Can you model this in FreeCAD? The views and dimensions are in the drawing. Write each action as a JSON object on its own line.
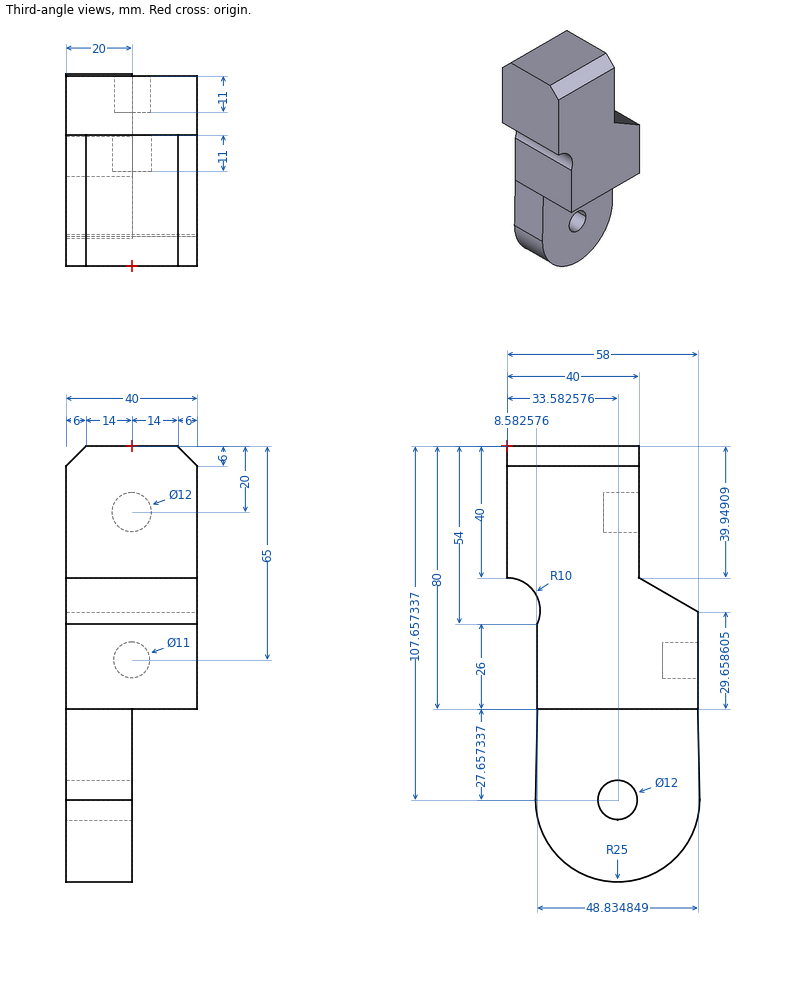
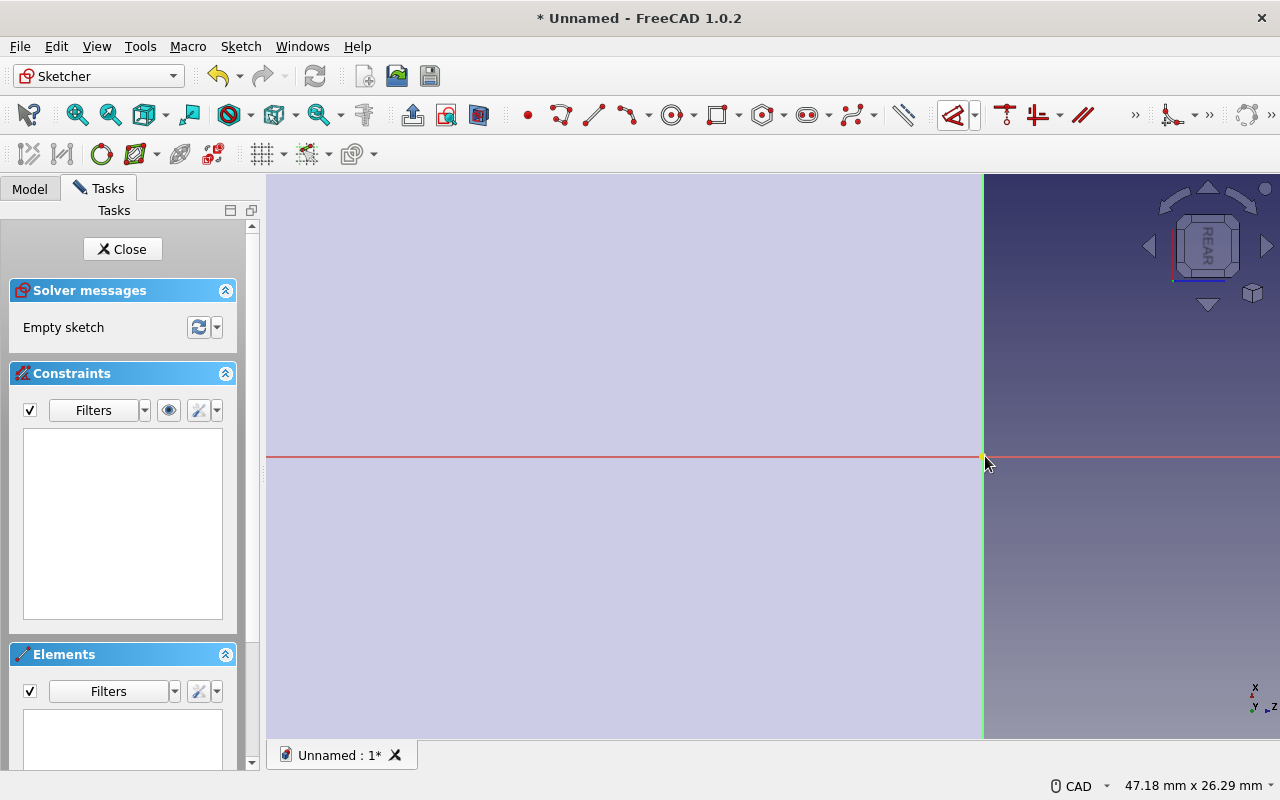
{"action": "key", "text": "g c"}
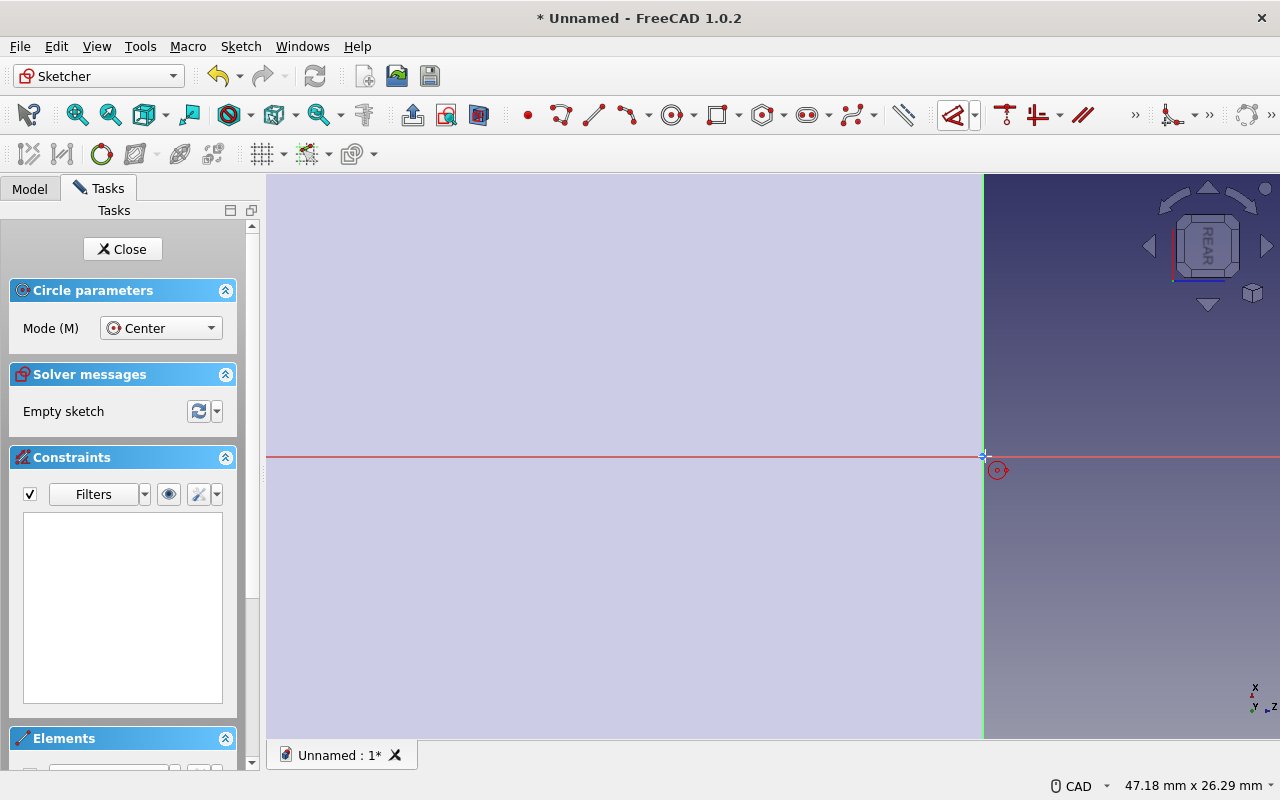
{"action": "left_click", "coordinate": [553, 456]}
{"action": "mouse_move", "coordinate": [644, 365]}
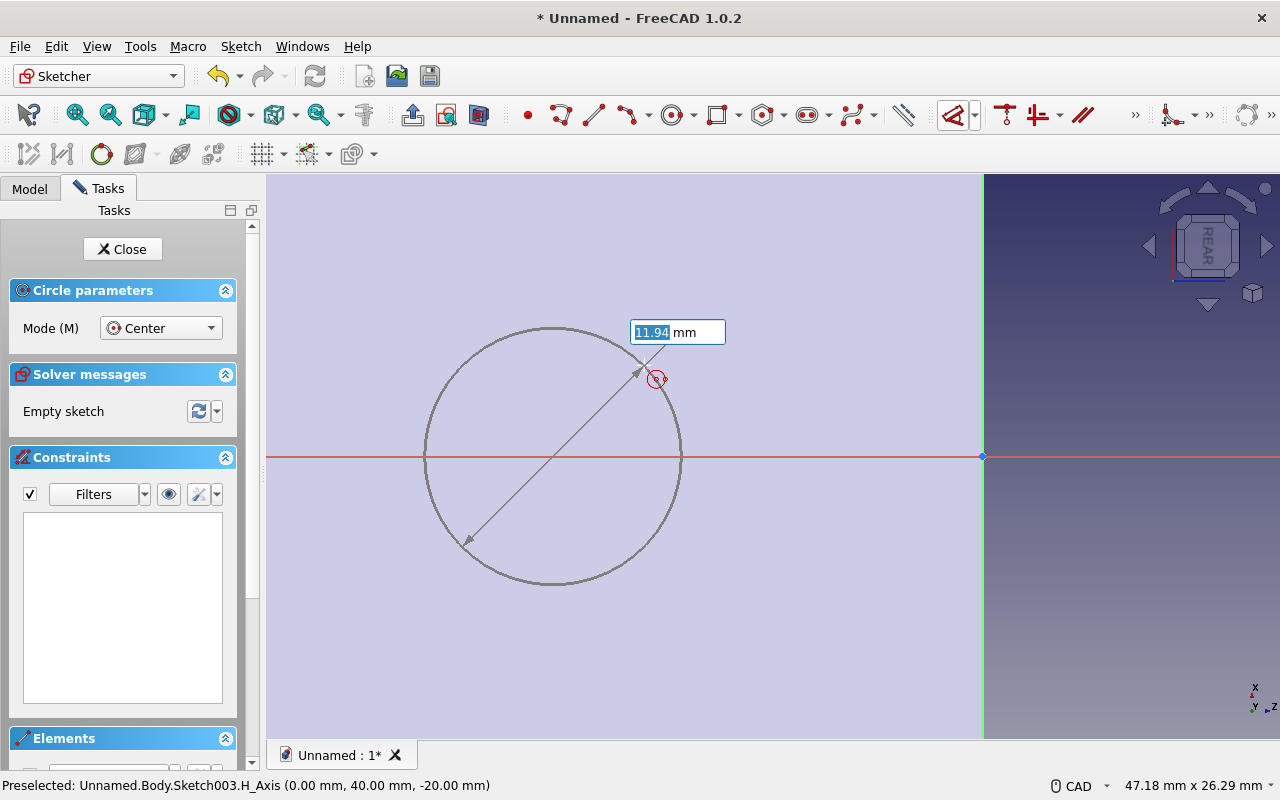
{"action": "type", "text": "12"}
{"action": "key", "text": "Return"}
{"action": "key", "text": "Escape"}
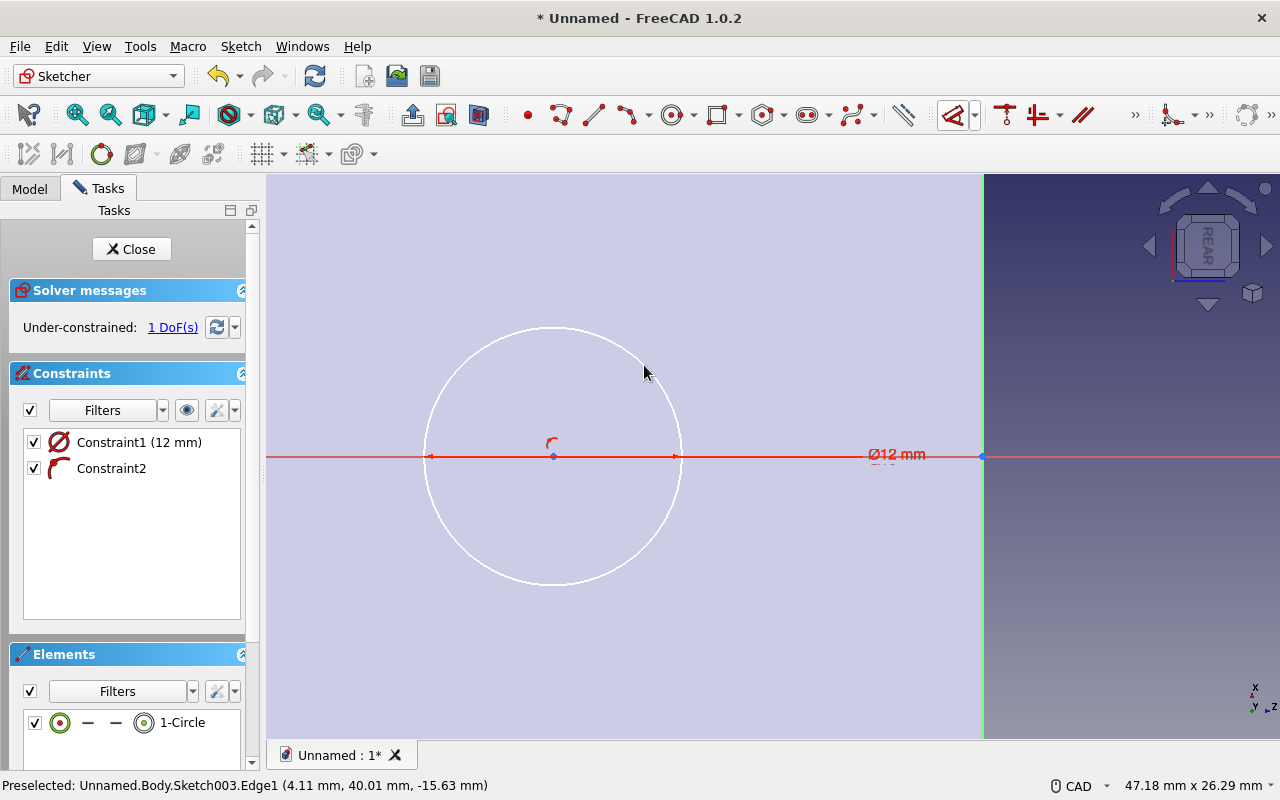
{"action": "left_click", "coordinate": [553, 456]}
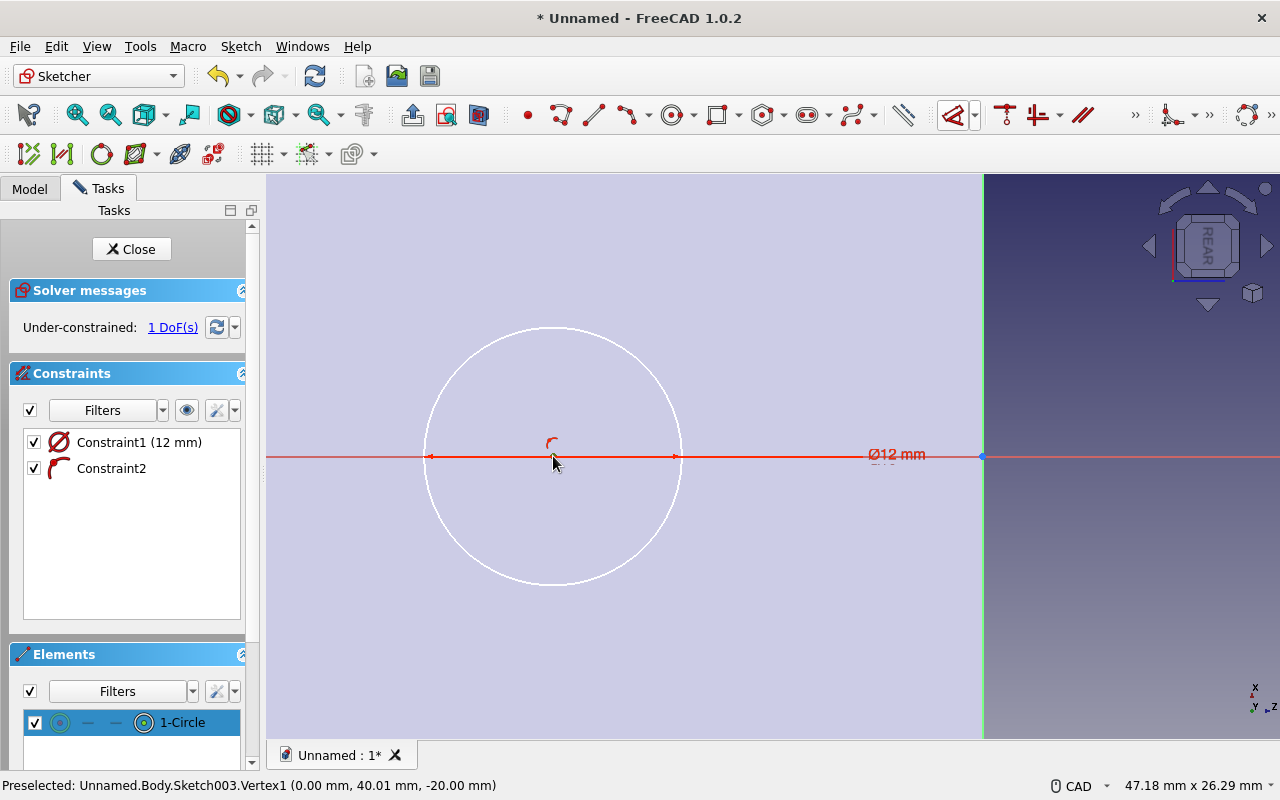
{"action": "left_click", "coordinate": [974, 116]}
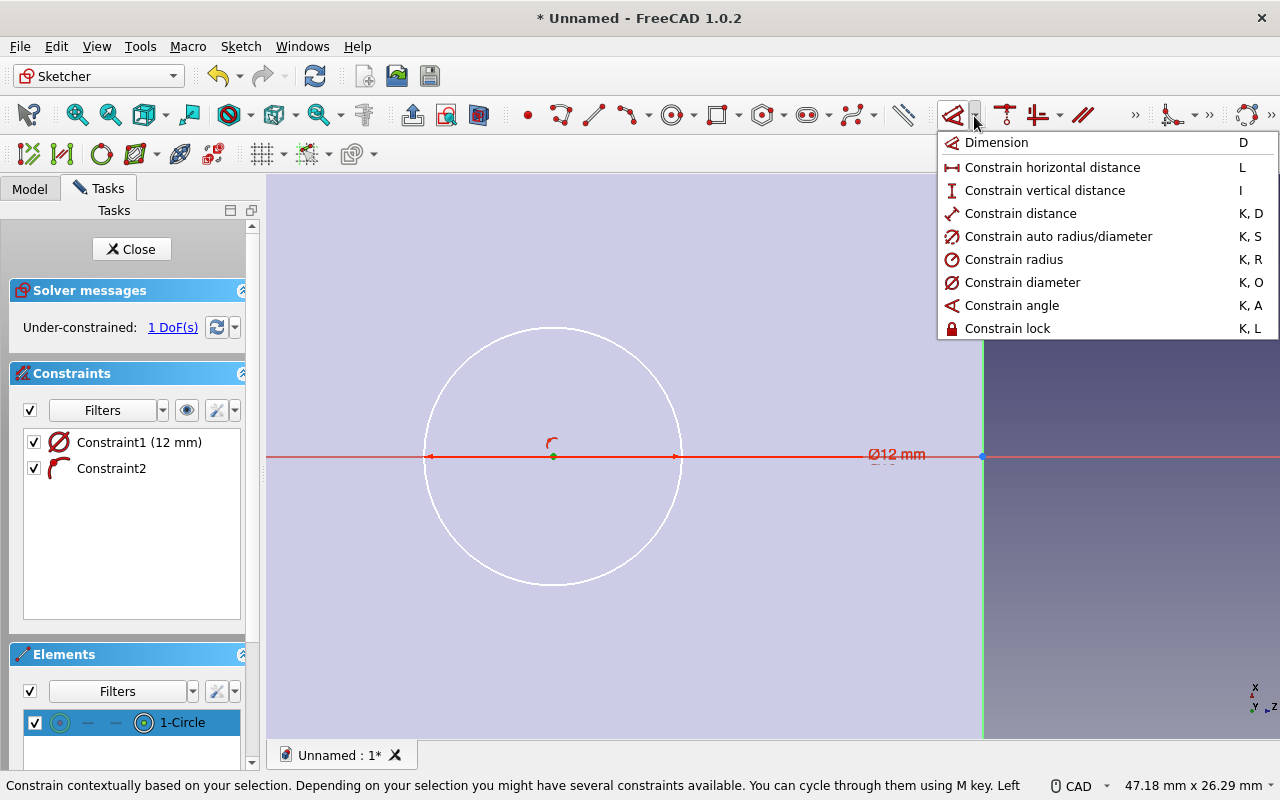
{"action": "left_click", "coordinate": [1108, 168]}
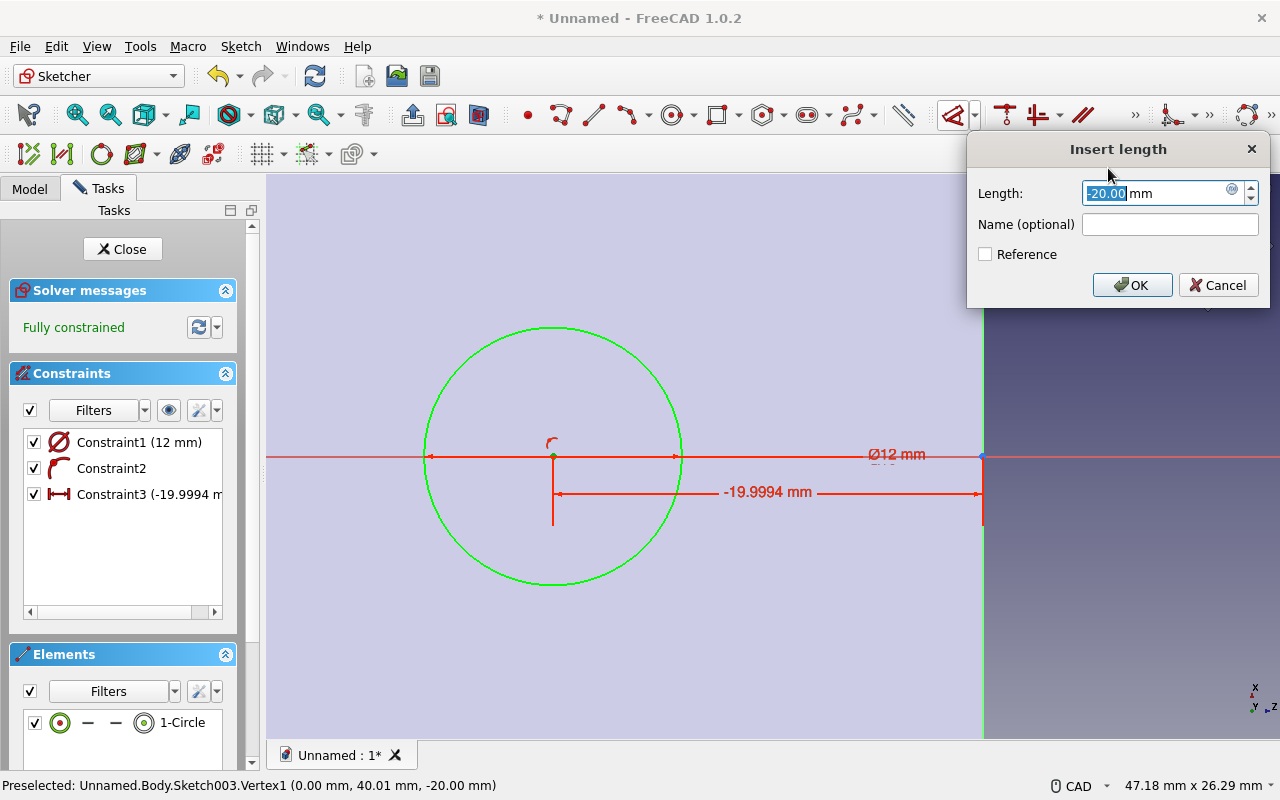
{"action": "type", "text": "-20"}
{"action": "key", "text": "Return"}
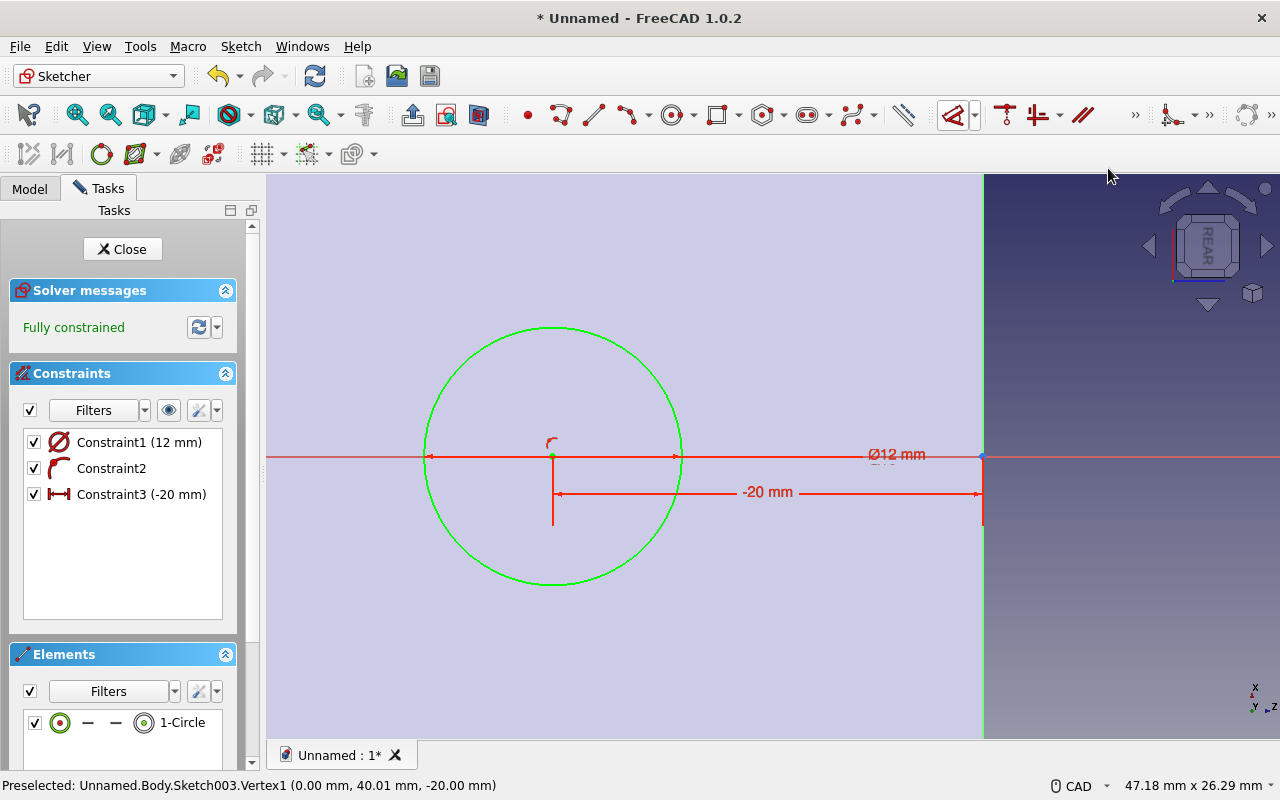
{"action": "left_click", "coordinate": [123, 249]}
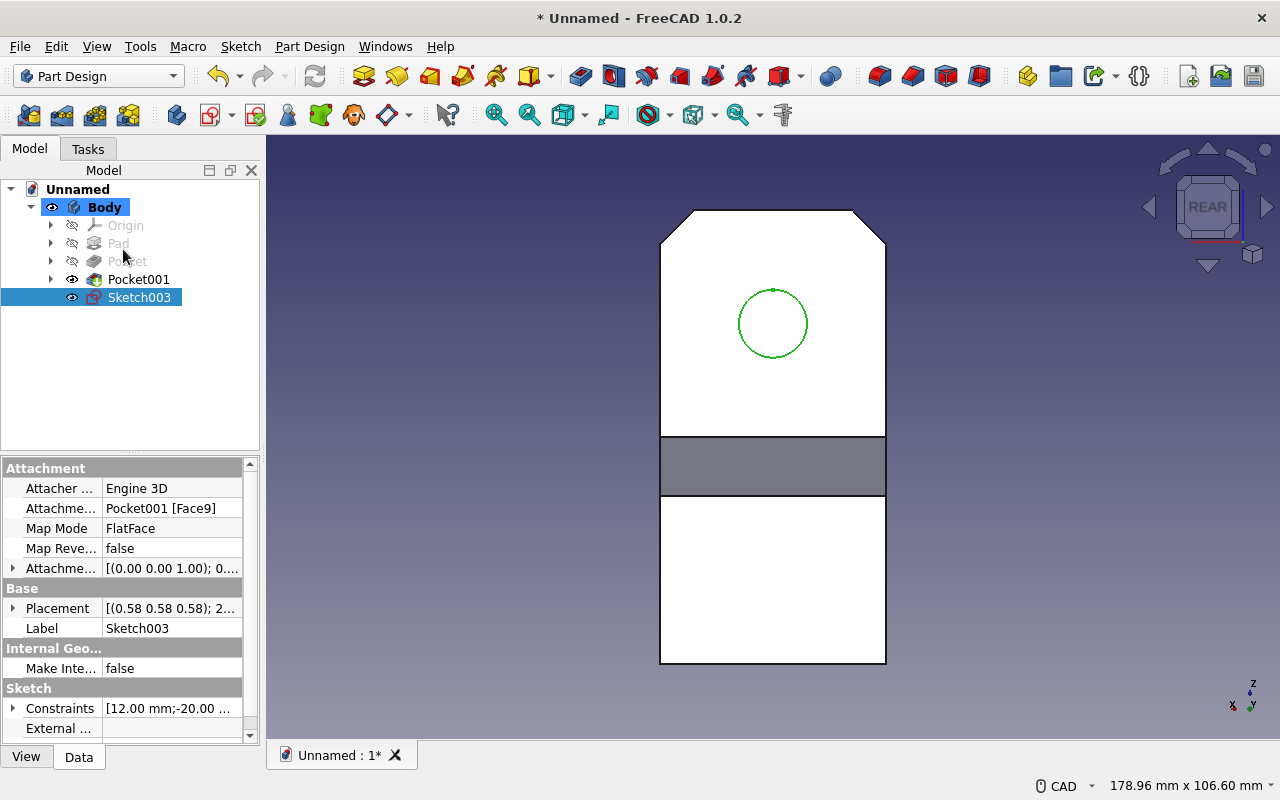
{"action": "left_click", "coordinate": [581, 76]}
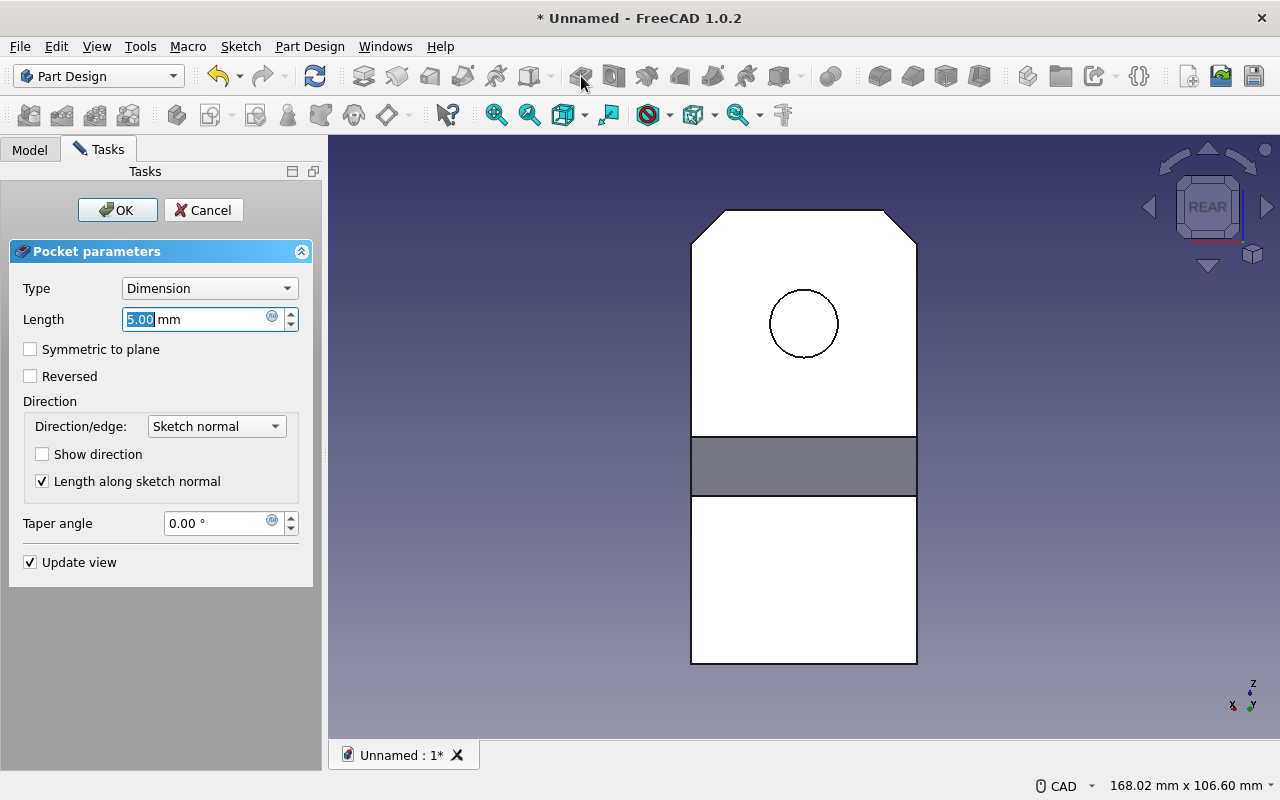
{"action": "type", "text": "11"}
{"action": "key", "text": "Tab"}